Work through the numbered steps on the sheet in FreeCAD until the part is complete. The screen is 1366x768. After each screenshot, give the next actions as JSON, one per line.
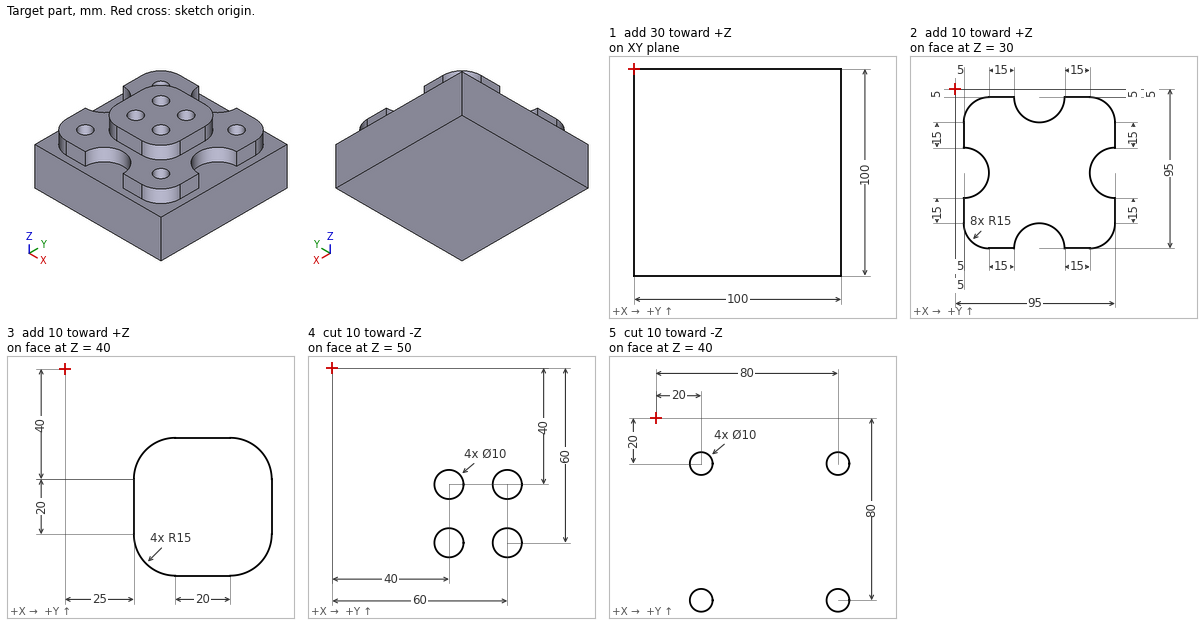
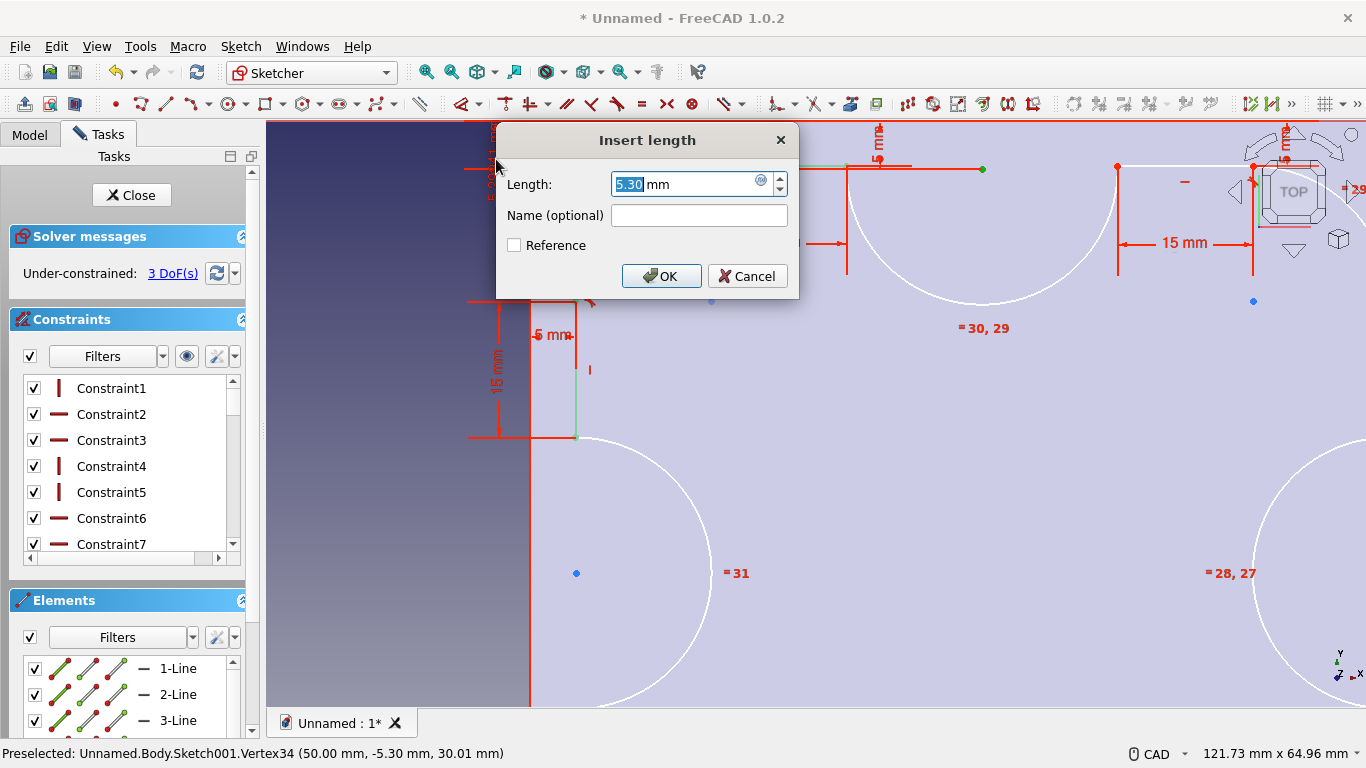
{"action": "type", "text": "5"}
{"action": "key", "text": "Return"}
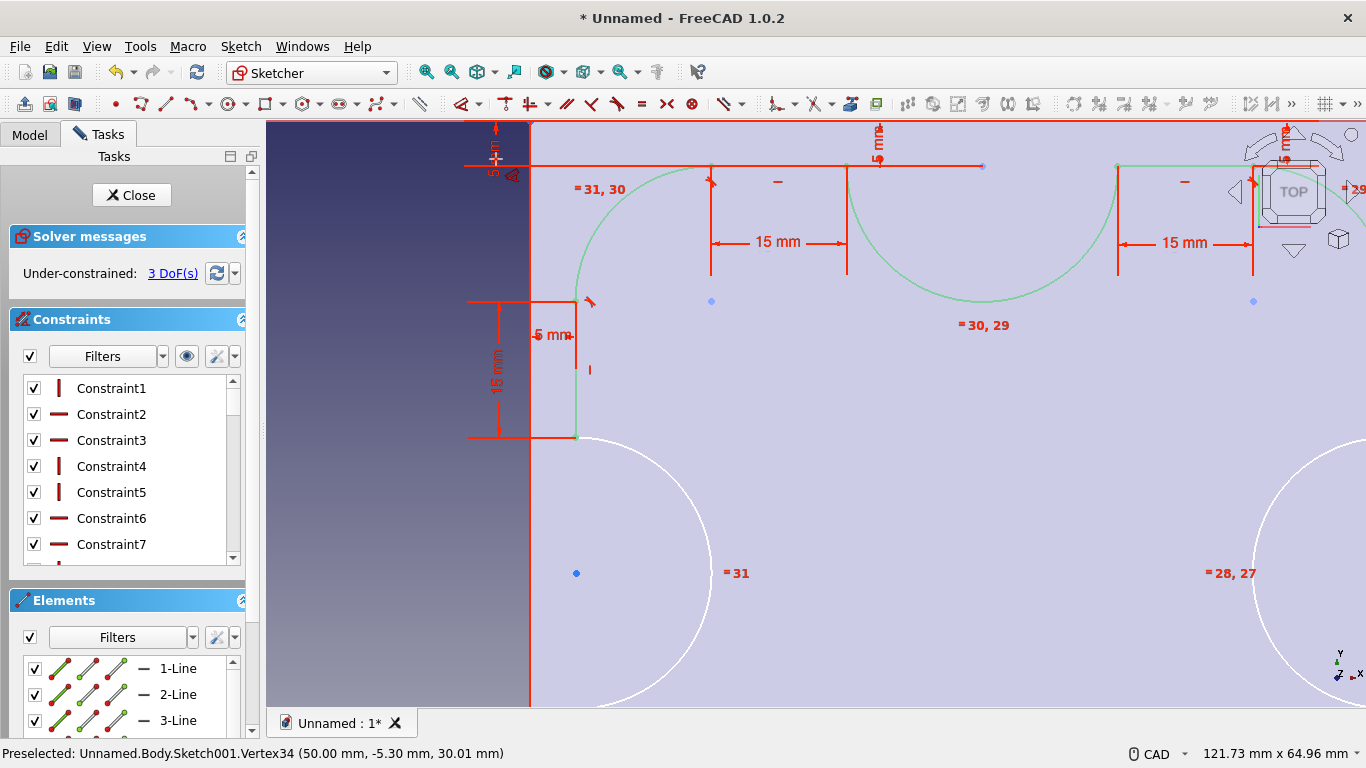
{"action": "left_click", "coordinate": [576, 573]}
{"action": "left_click", "coordinate": [553, 607]}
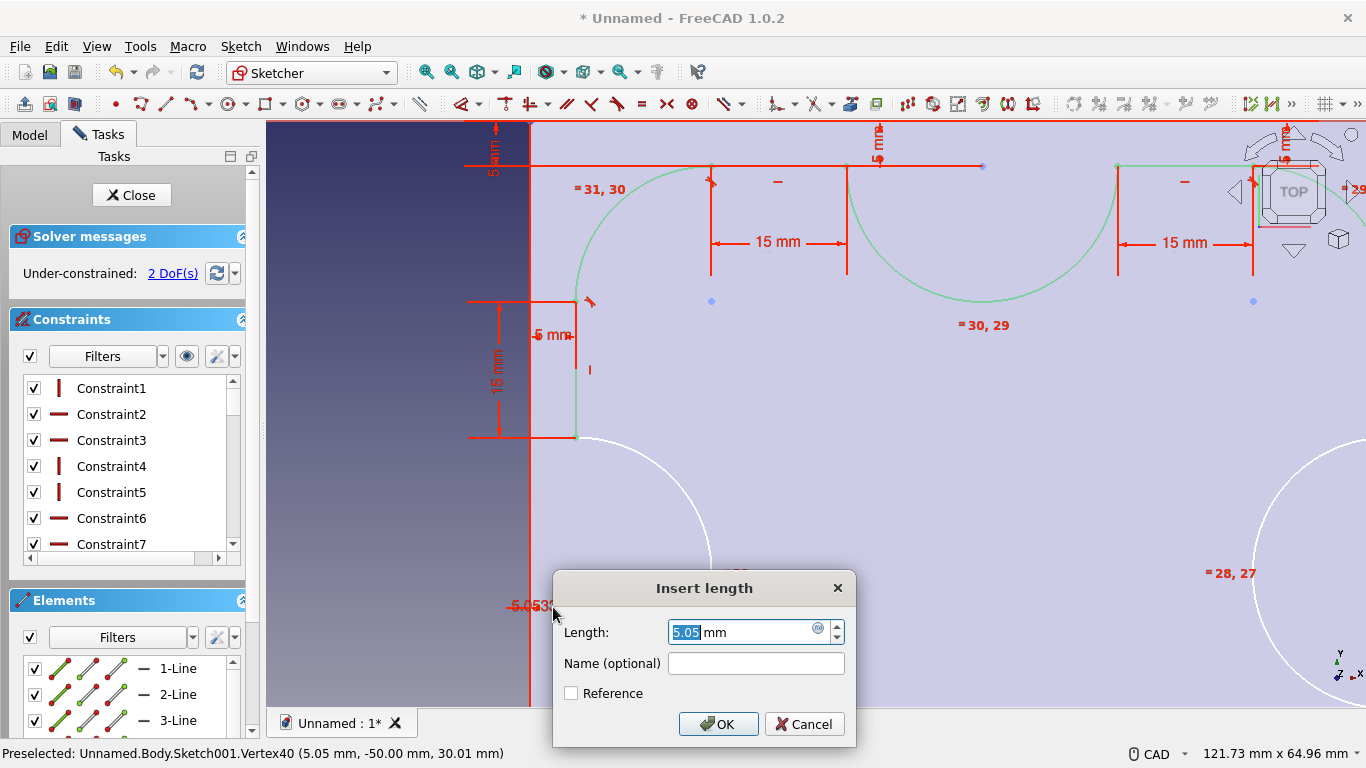
{"action": "type", "text": "5"}
{"action": "key", "text": "Return"}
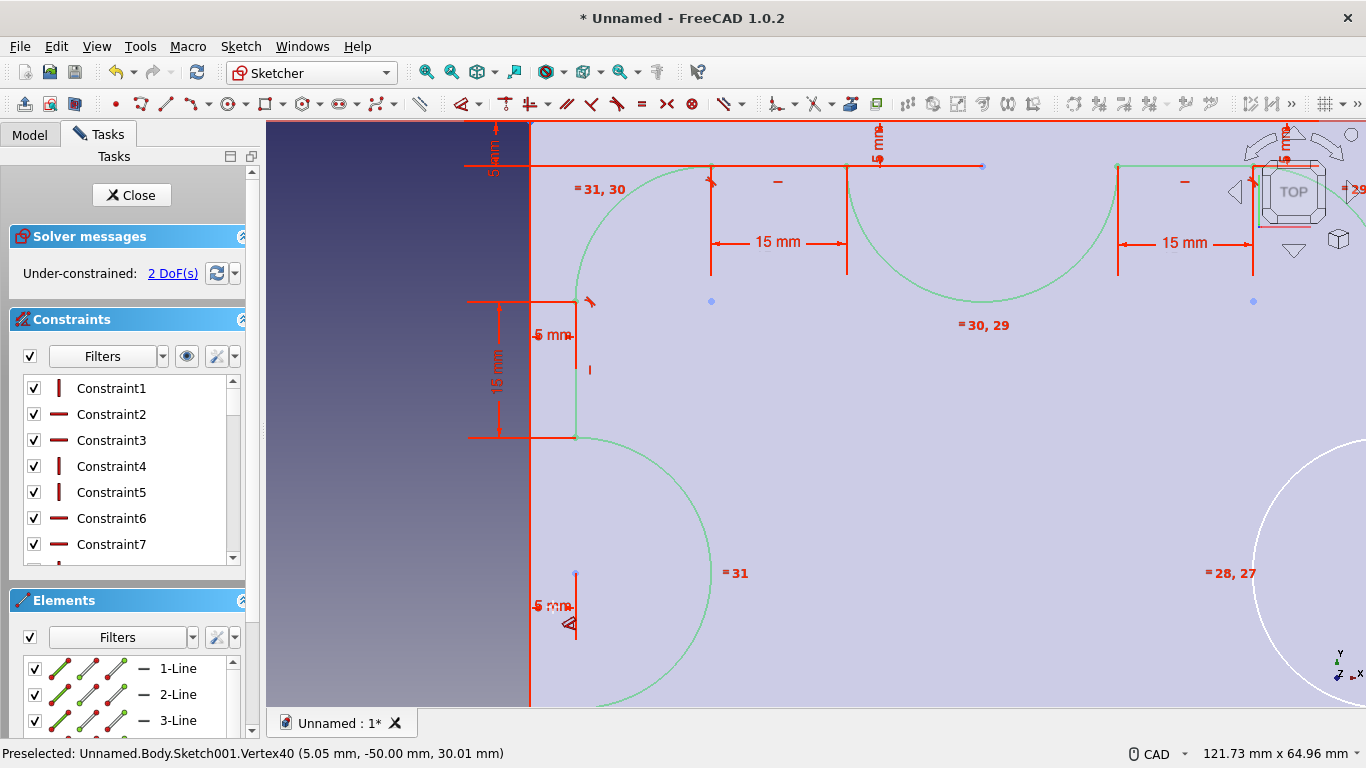
{"action": "scroll", "coordinate": [574, 302], "scroll_direction": "down", "scroll_amount": 4}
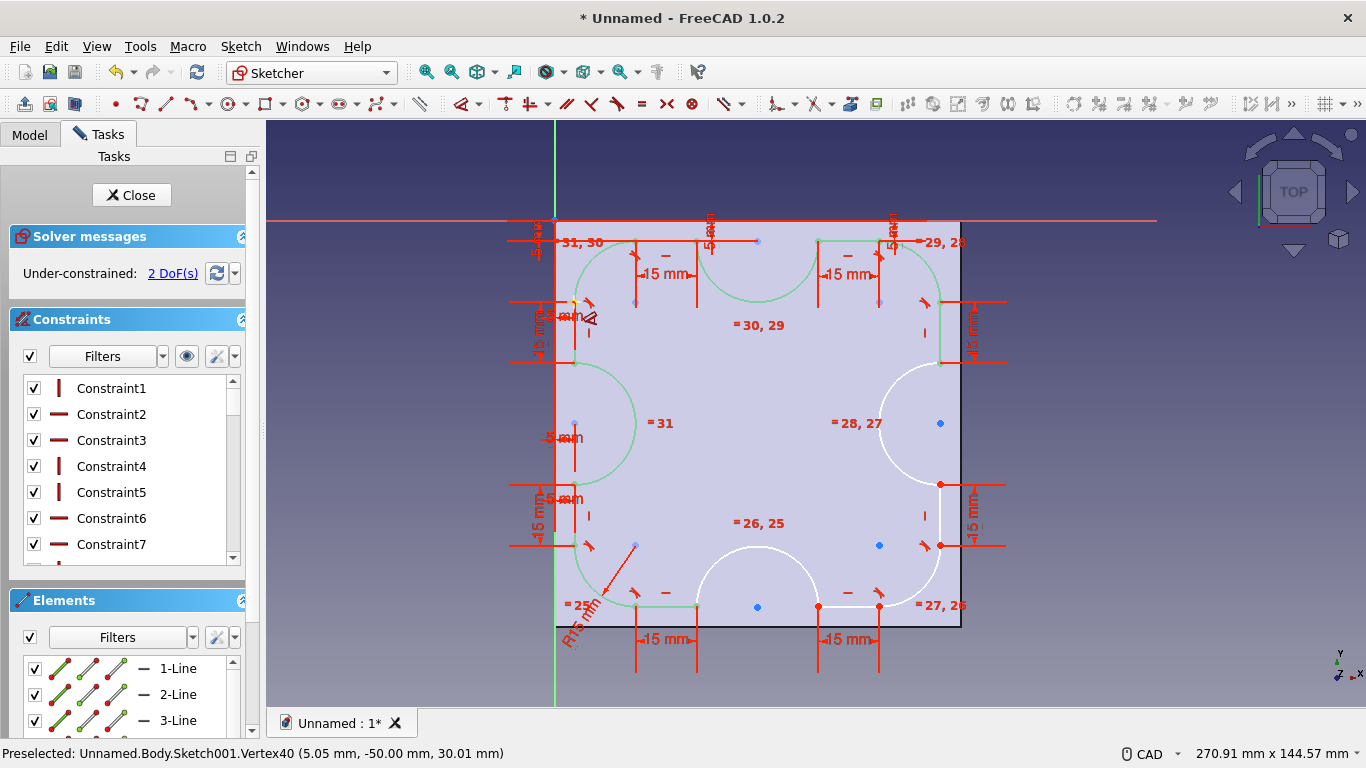
{"action": "left_click", "coordinate": [758, 607]}
{"action": "left_click", "coordinate": [521, 414]}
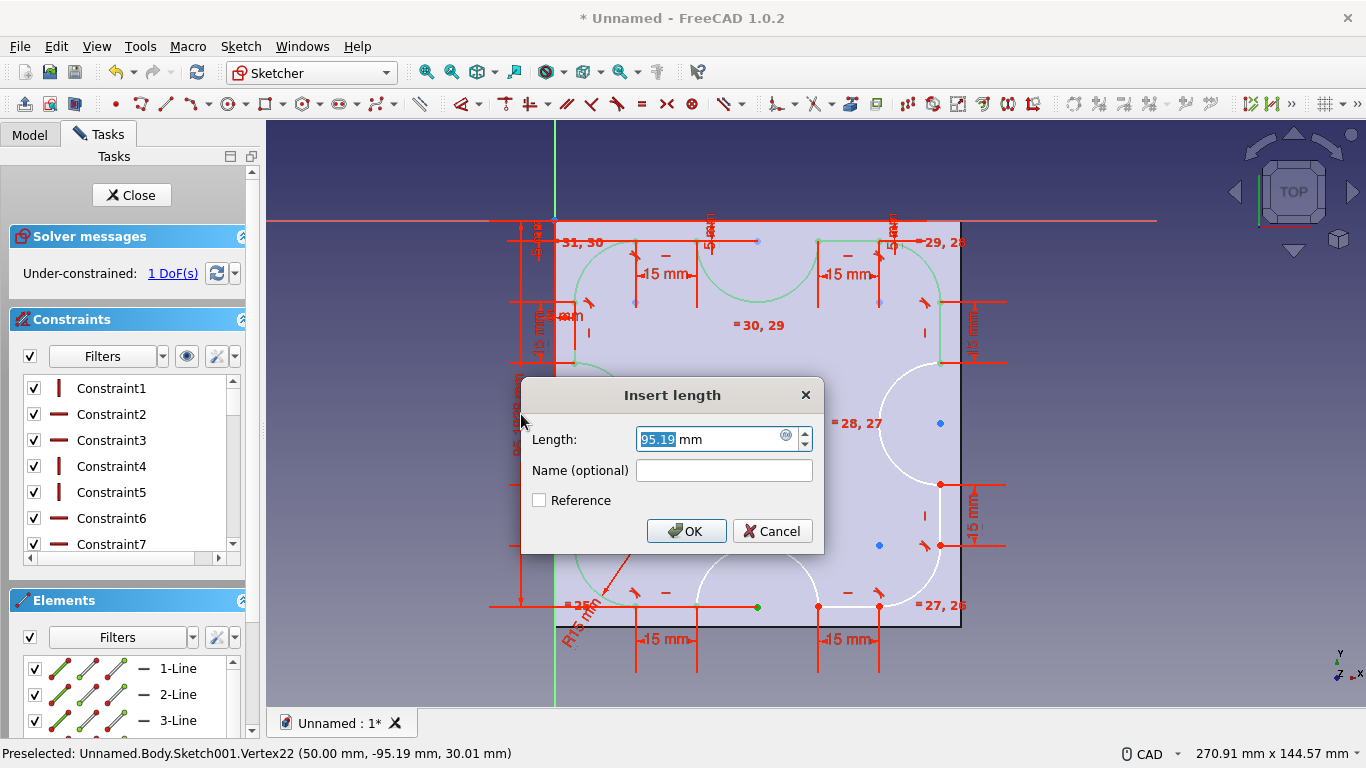
{"action": "type", "text": "95"}
{"action": "key", "text": "Return"}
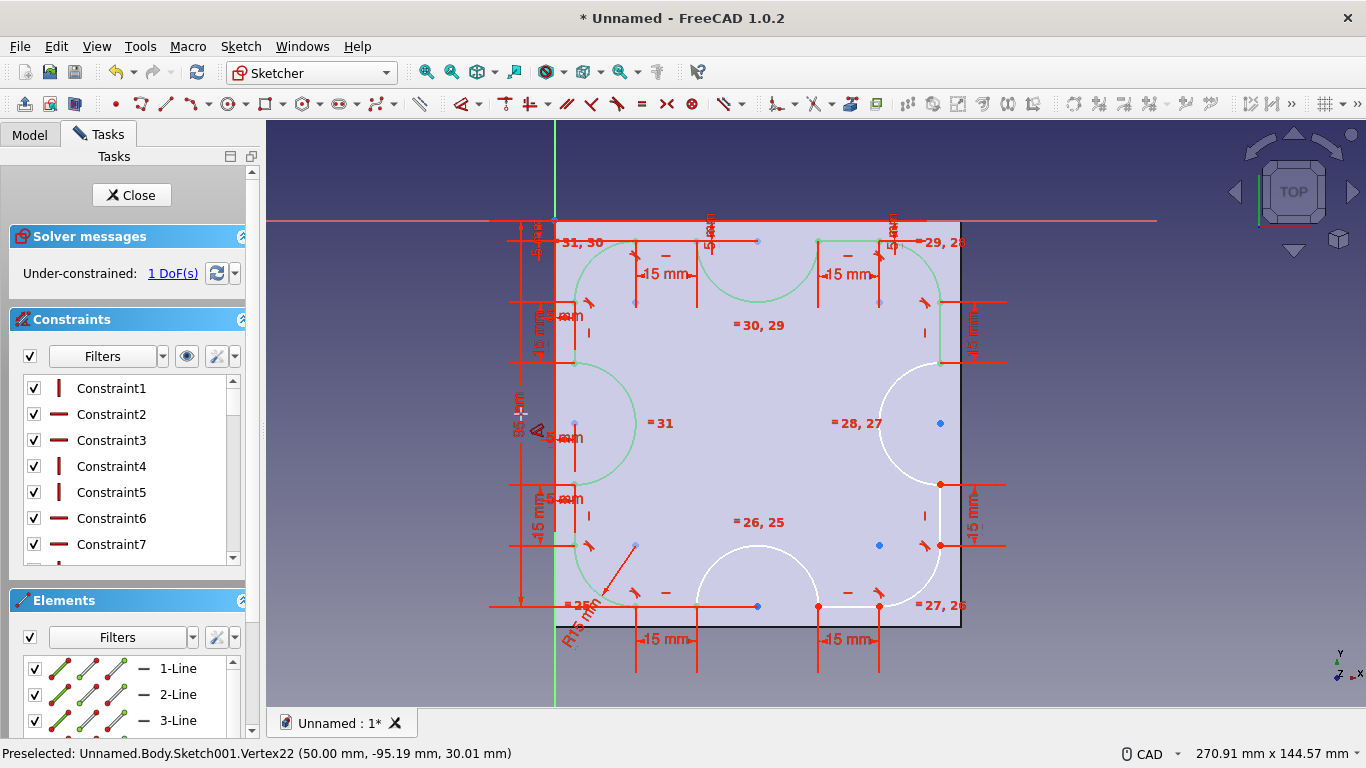
{"action": "left_click", "coordinate": [940, 424]}
{"action": "left_click", "coordinate": [747, 187]}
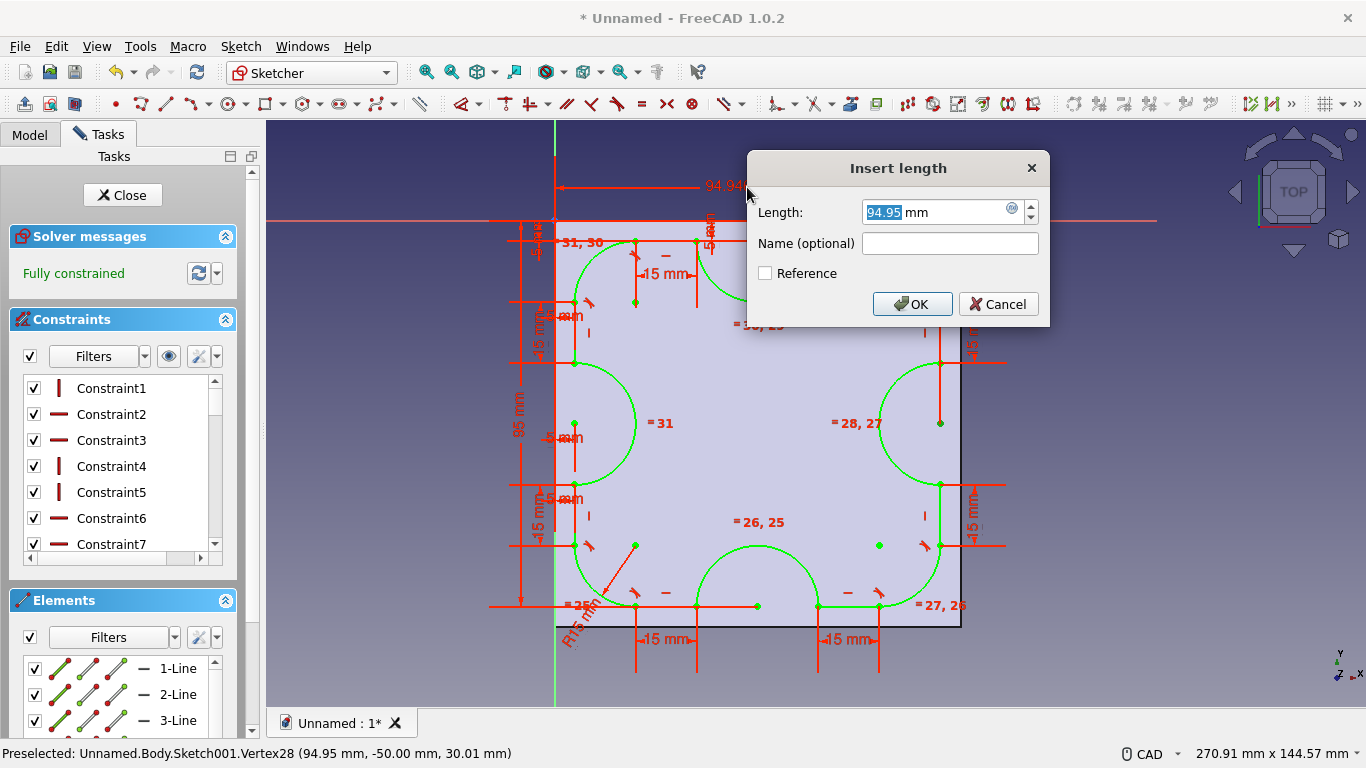
{"action": "type", "text": "95"}
{"action": "key", "text": "Return"}
{"action": "key", "text": "Escape"}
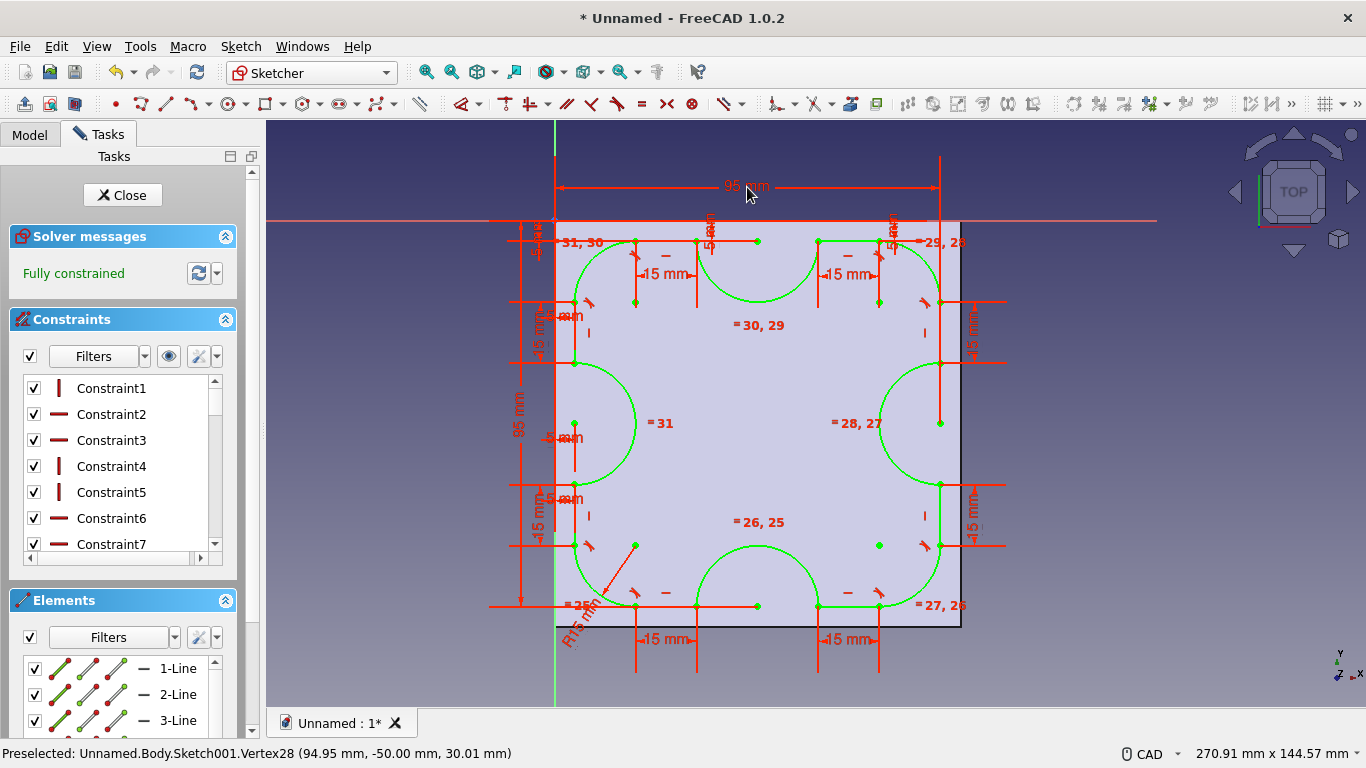
{"action": "left_click", "coordinate": [123, 195]}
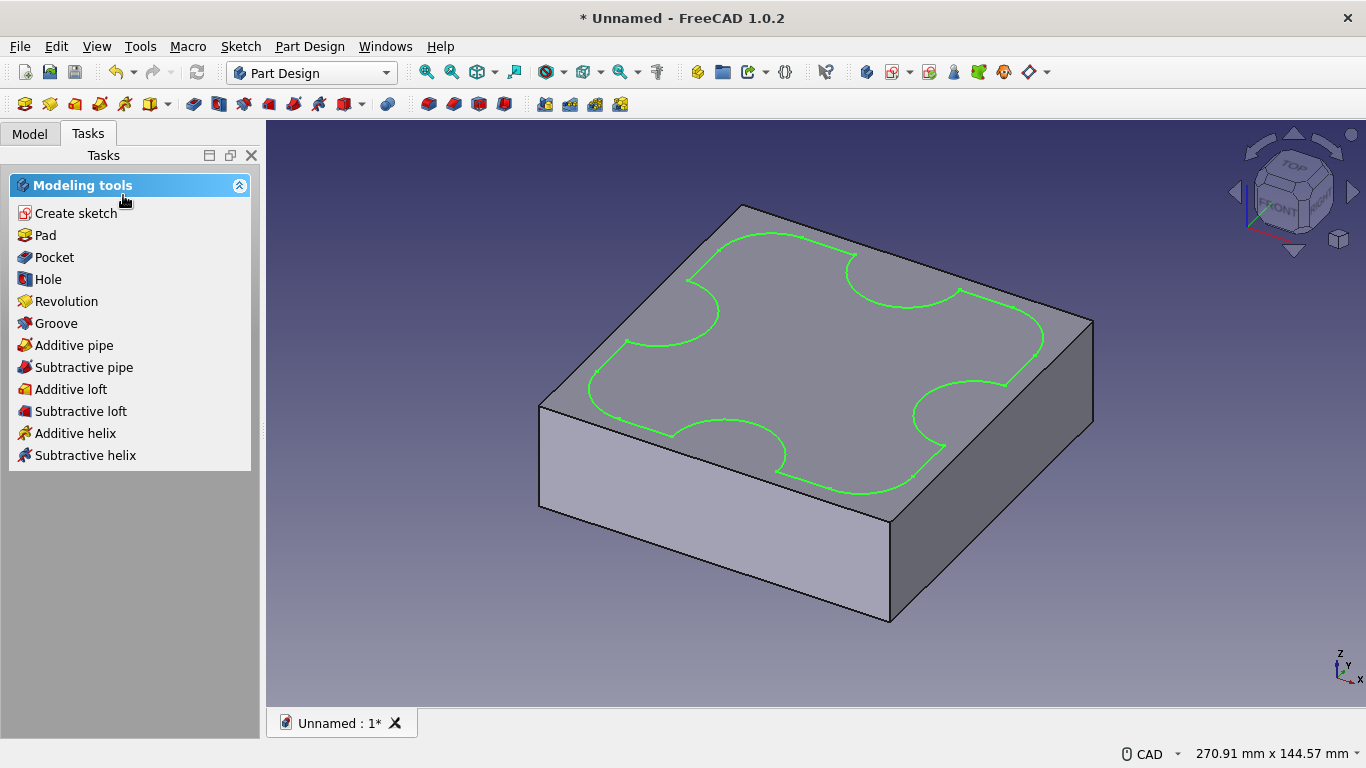
{"action": "left_click", "coordinate": [25, 104]}